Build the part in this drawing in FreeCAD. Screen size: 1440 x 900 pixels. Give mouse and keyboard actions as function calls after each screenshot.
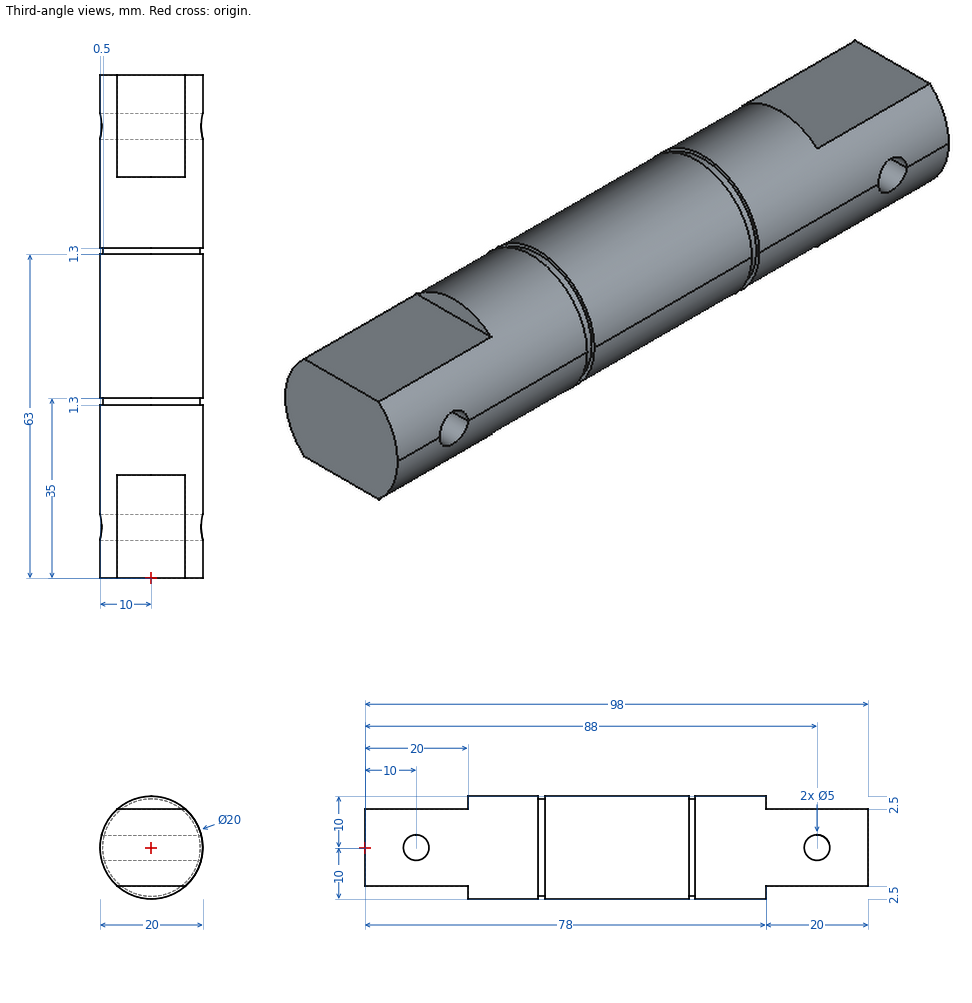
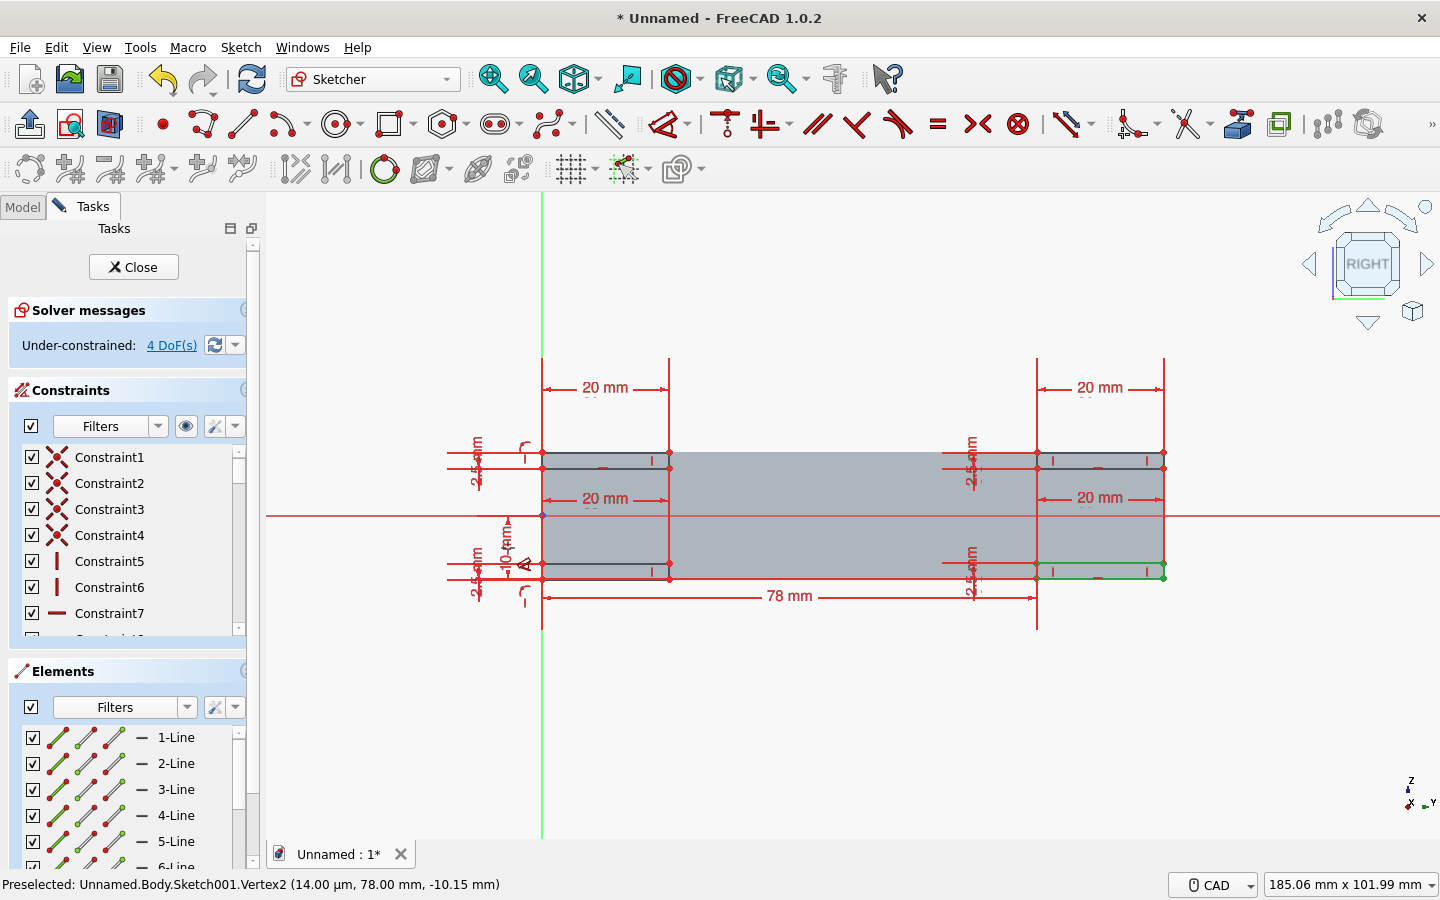
click(1037, 453)
click(790, 419)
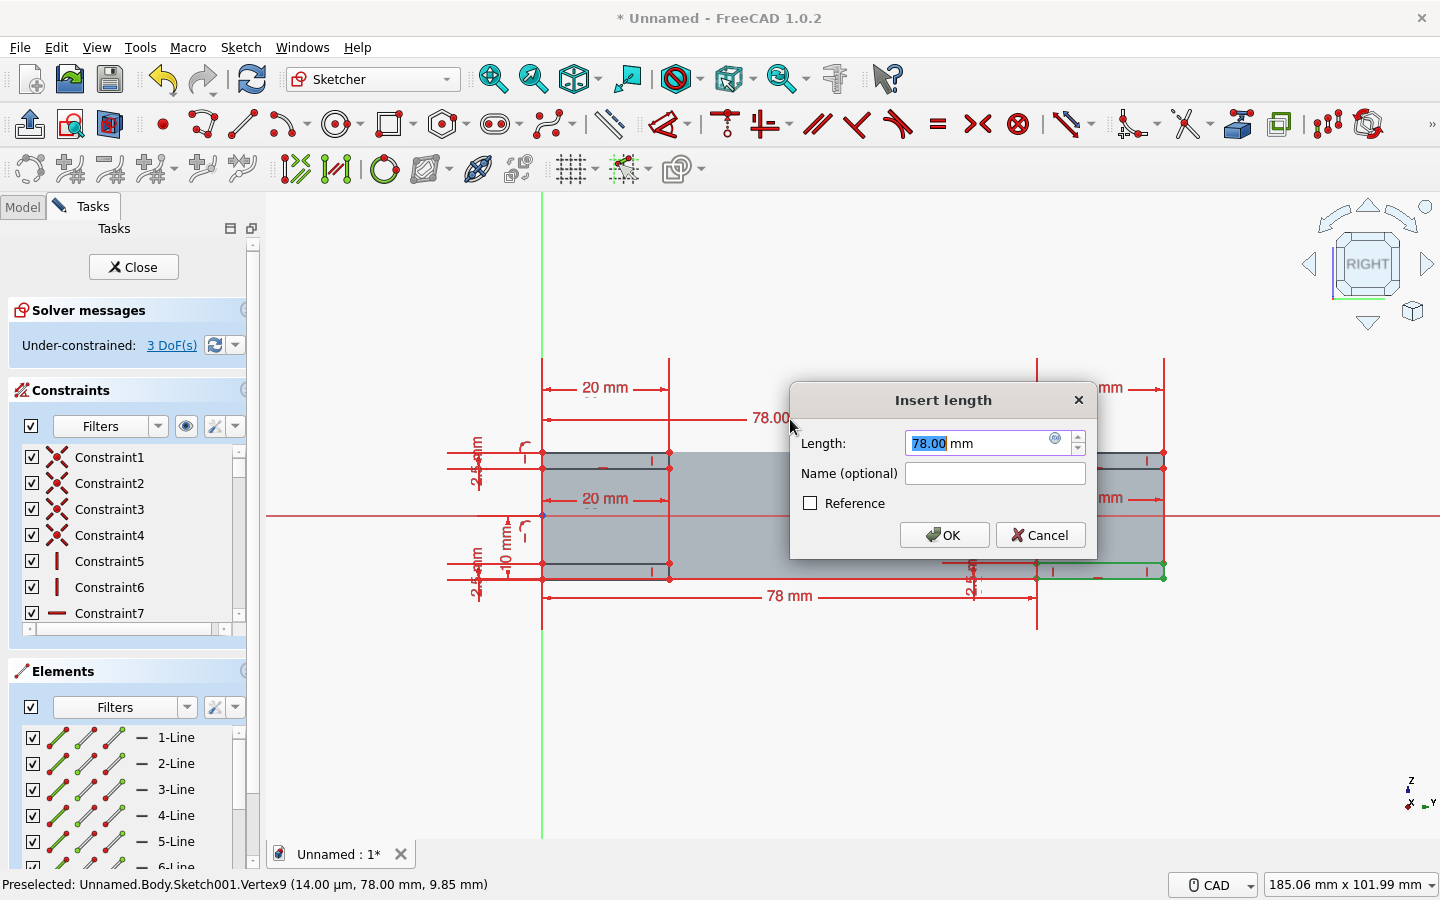
text(78)
key(Return)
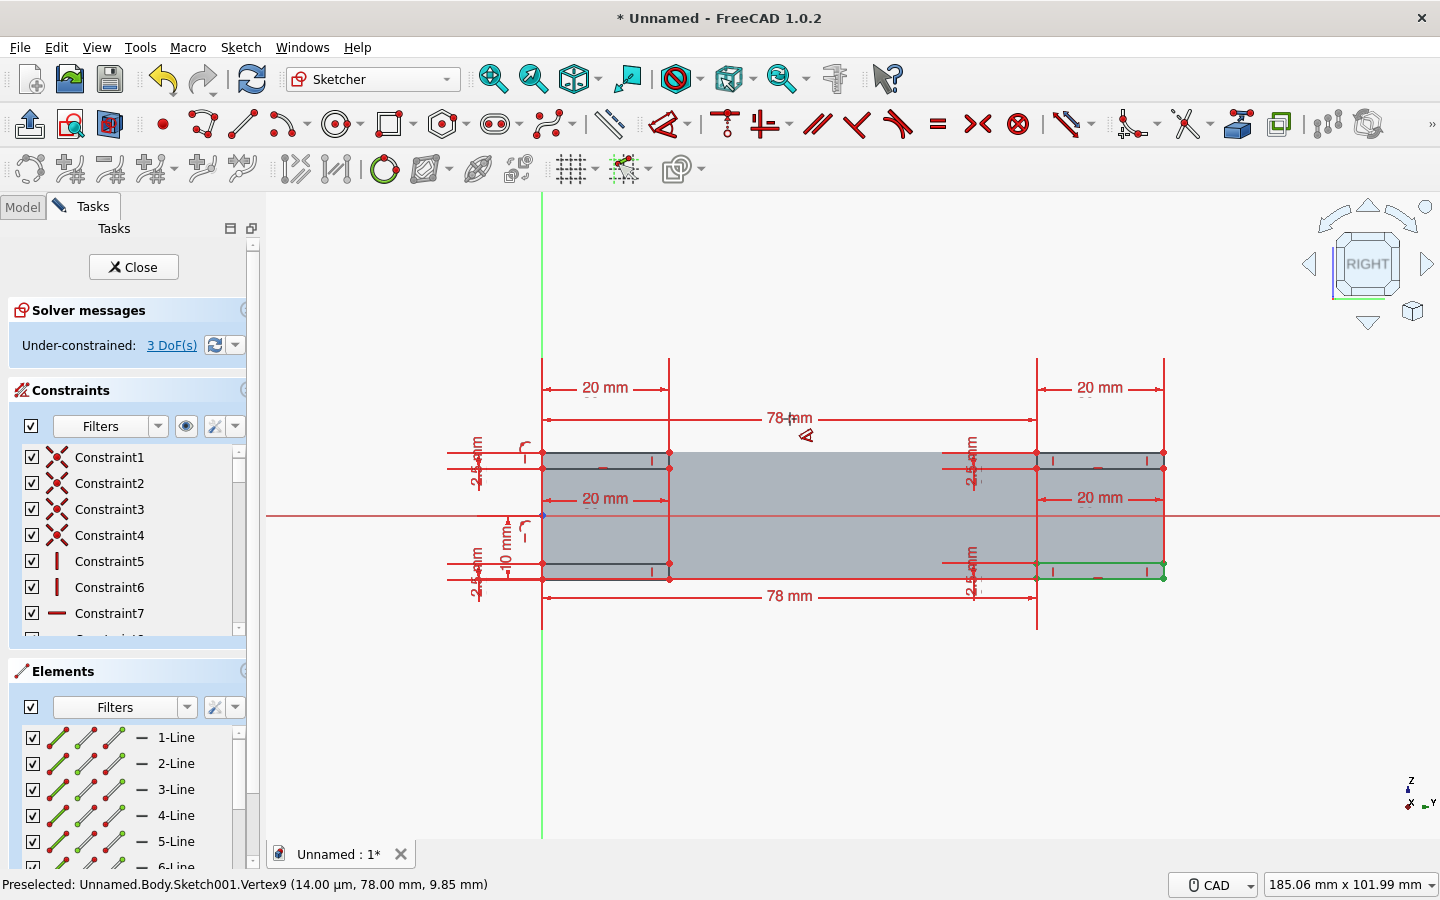
click(1037, 453)
click(508, 484)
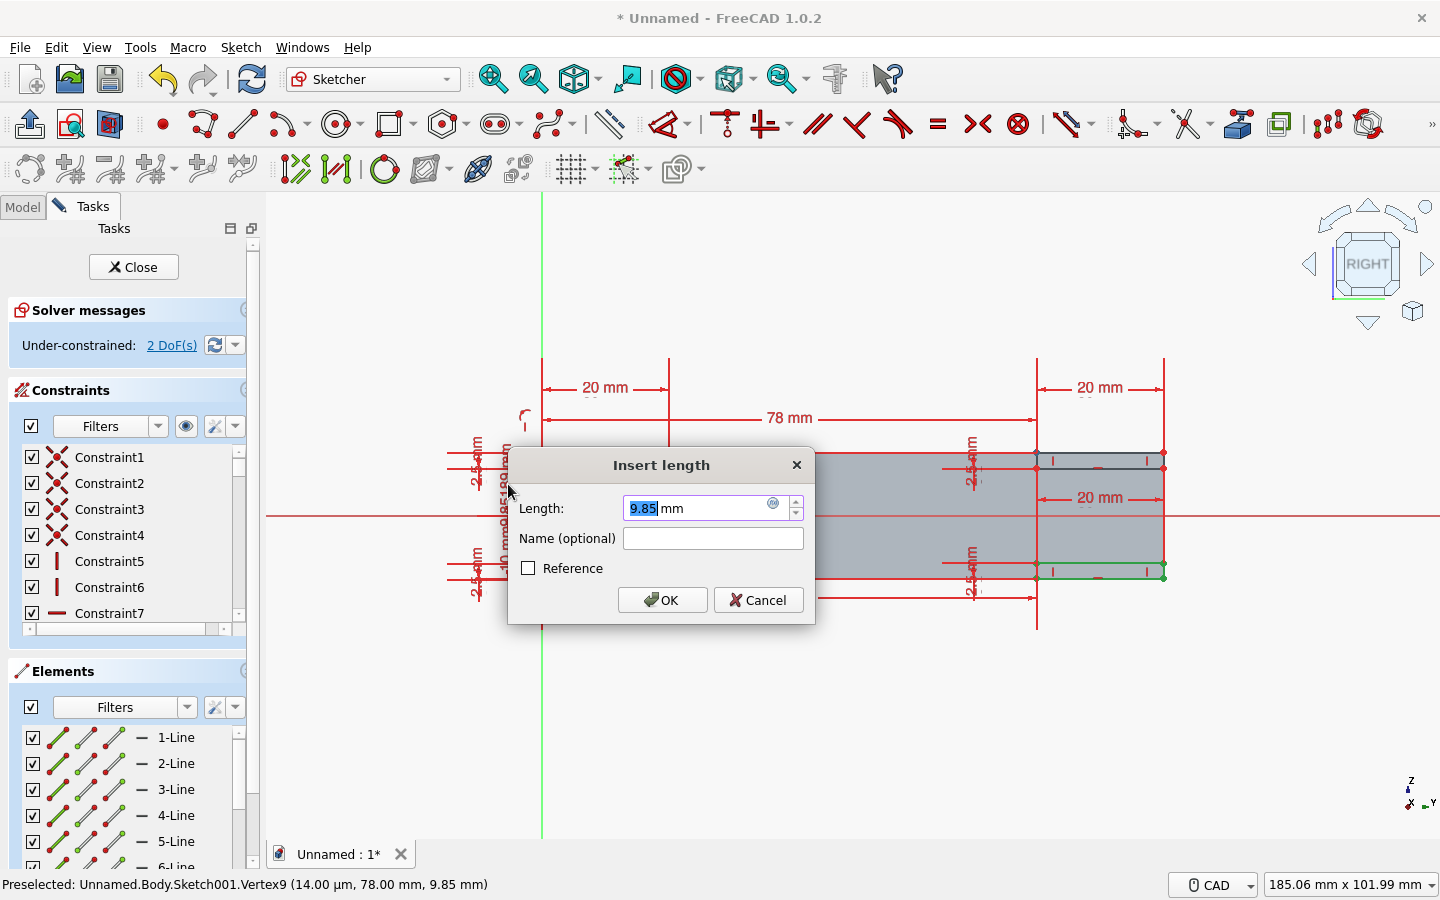
text(10)
key(Return)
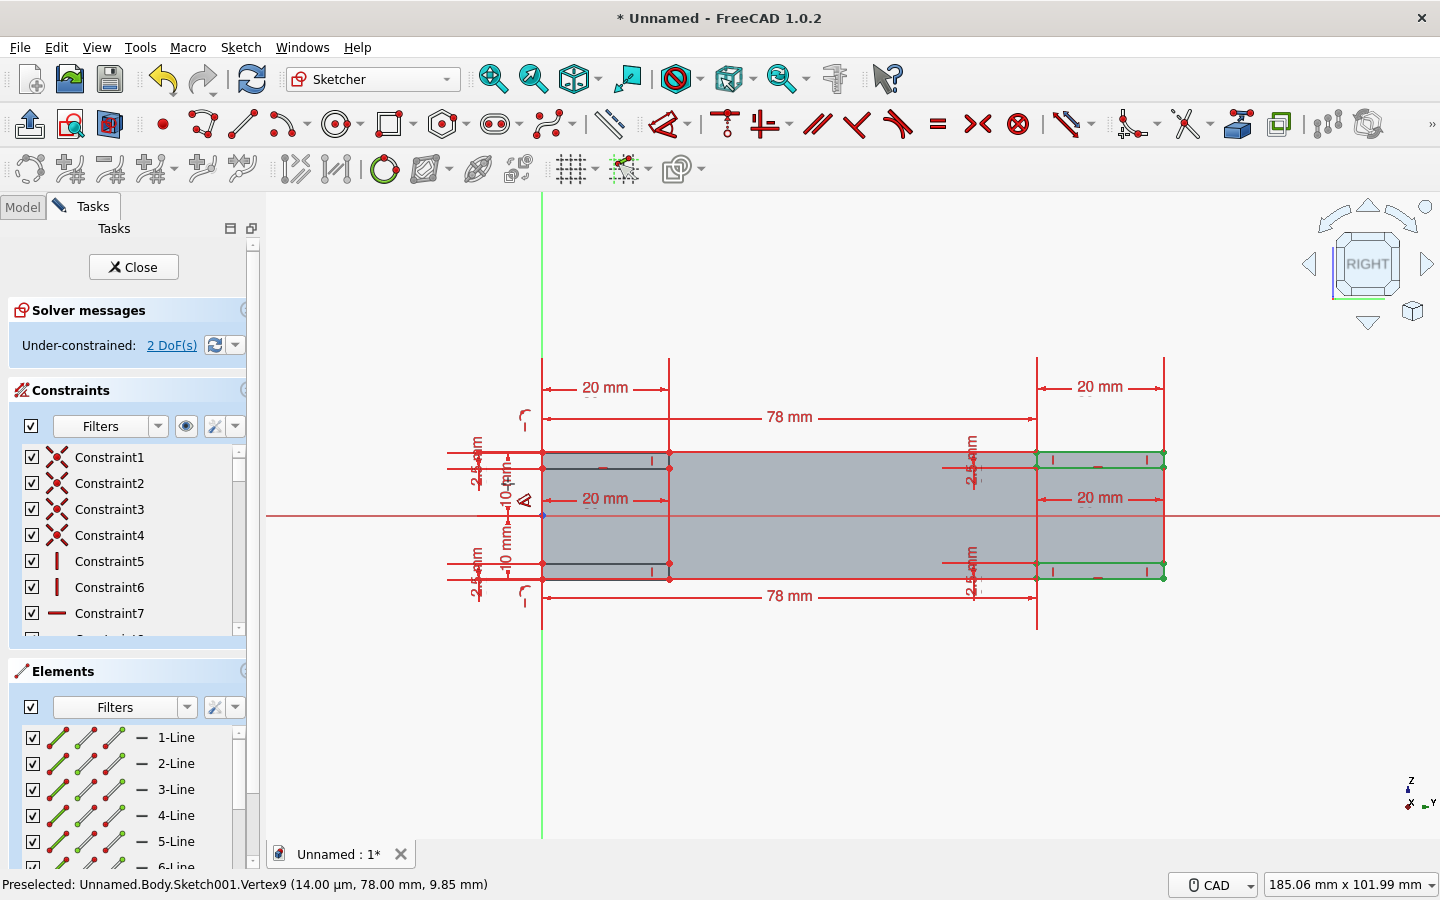
click(542, 453)
click(508, 462)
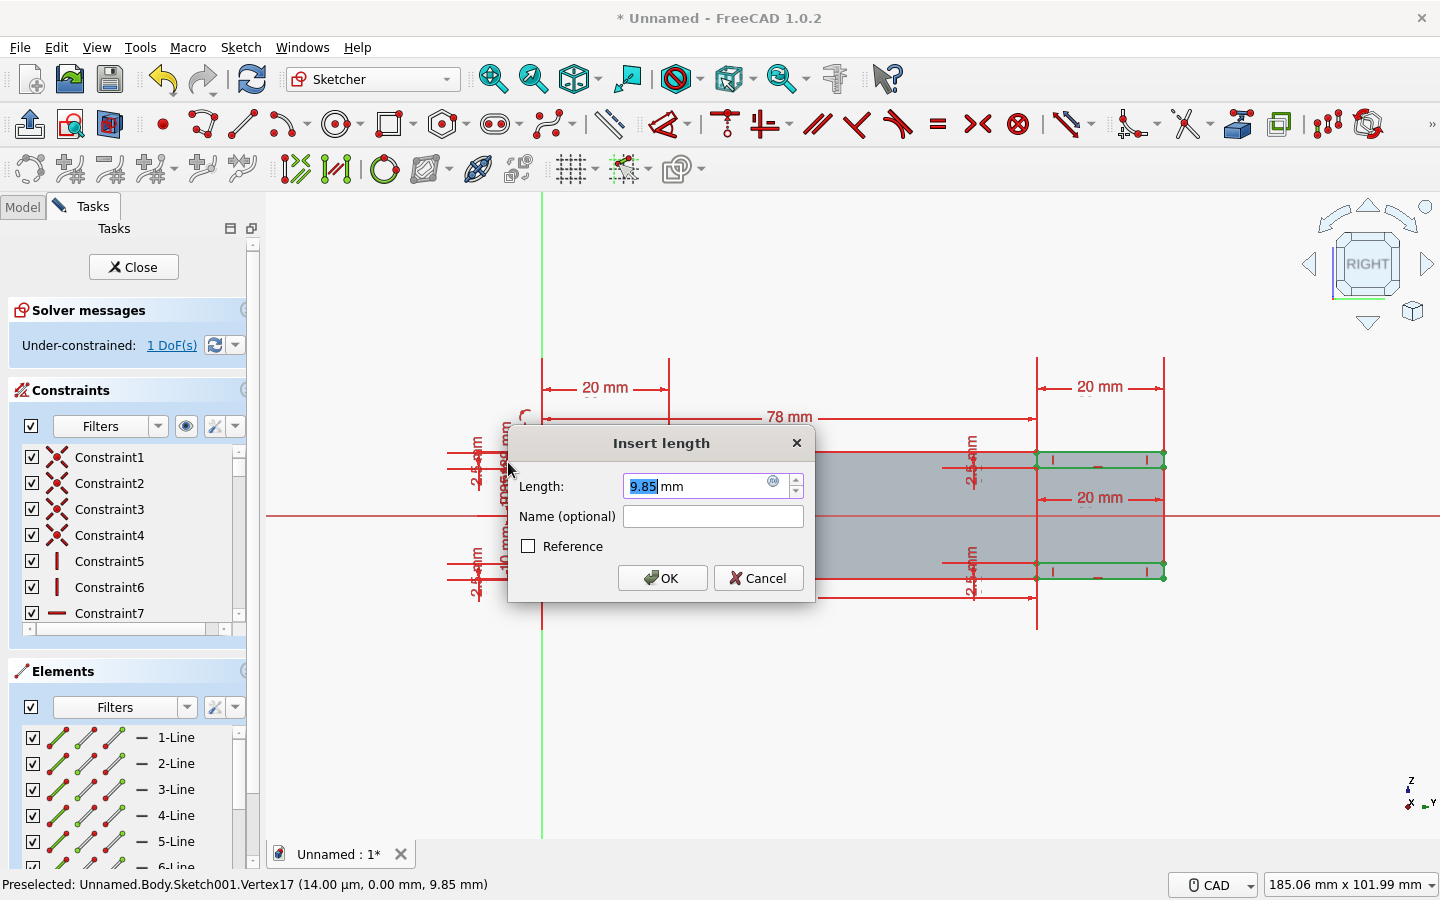
text(10)
key(Return)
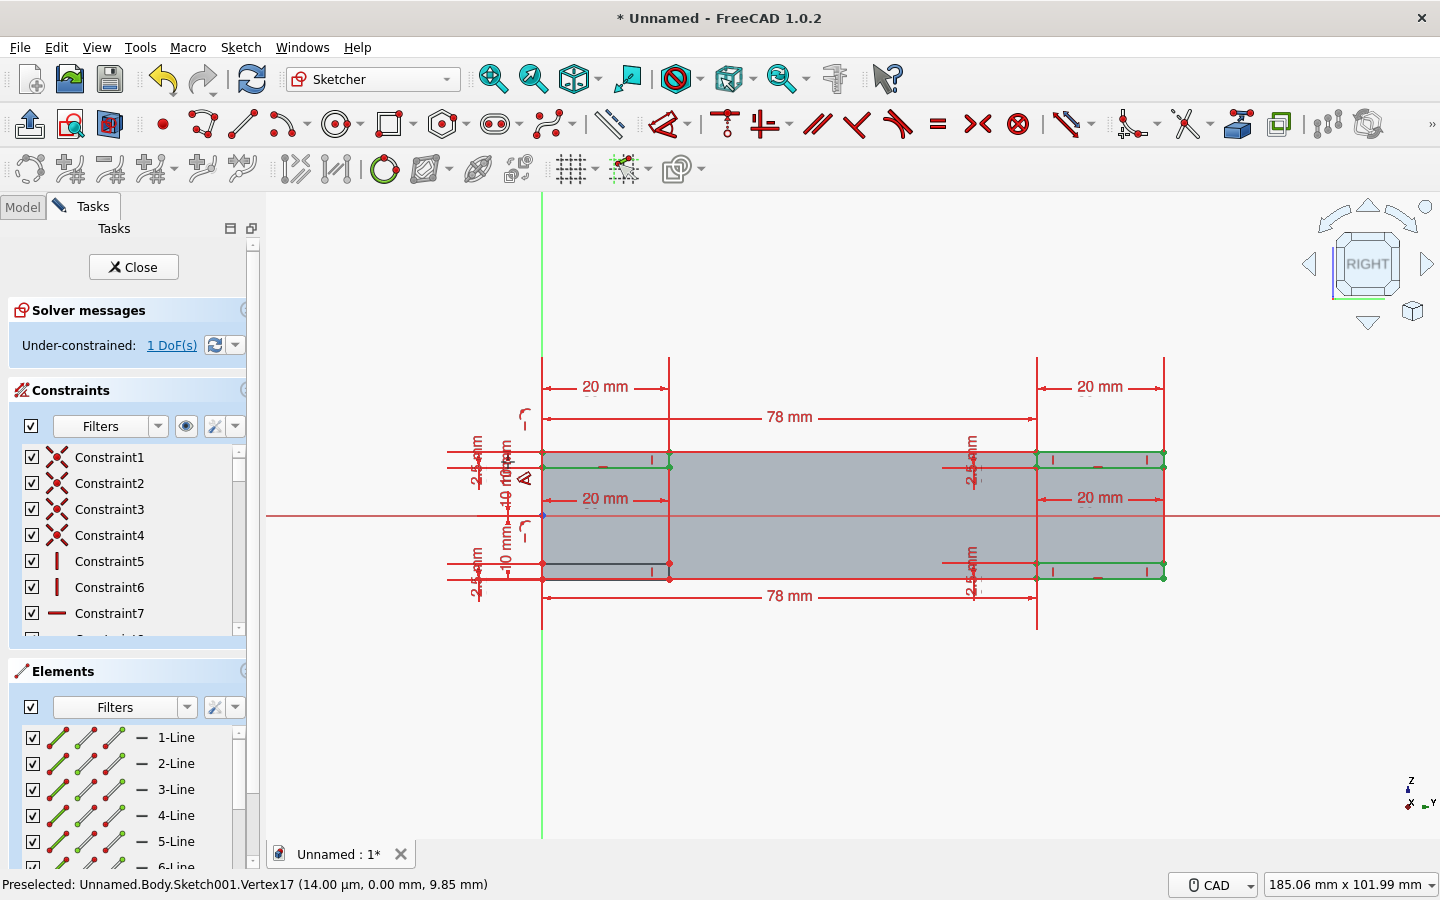
click(542, 580)
click(508, 570)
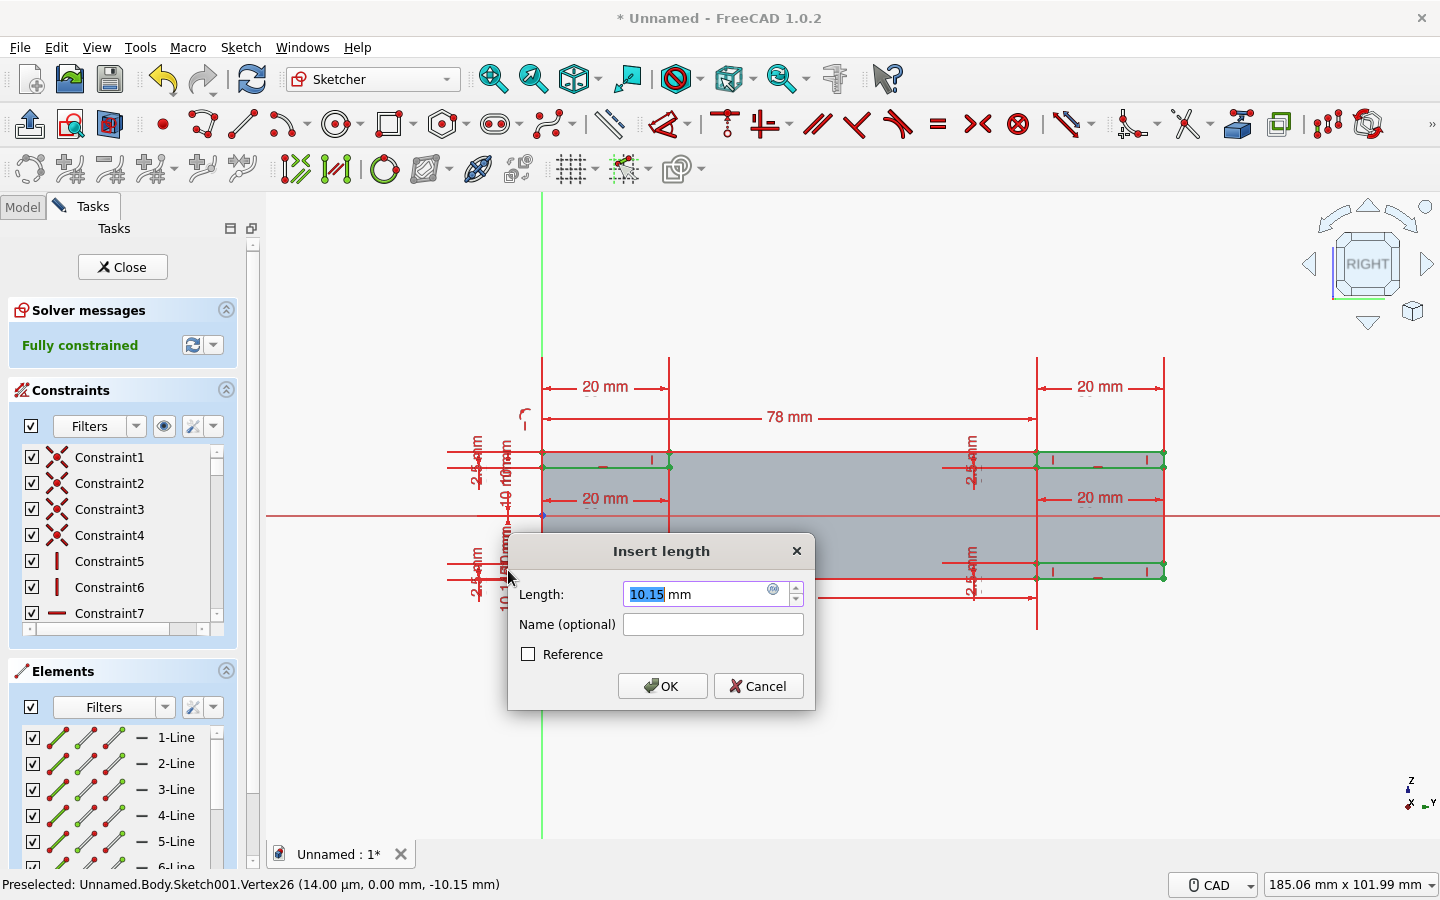
text(10)
key(Return)
key(Escape)